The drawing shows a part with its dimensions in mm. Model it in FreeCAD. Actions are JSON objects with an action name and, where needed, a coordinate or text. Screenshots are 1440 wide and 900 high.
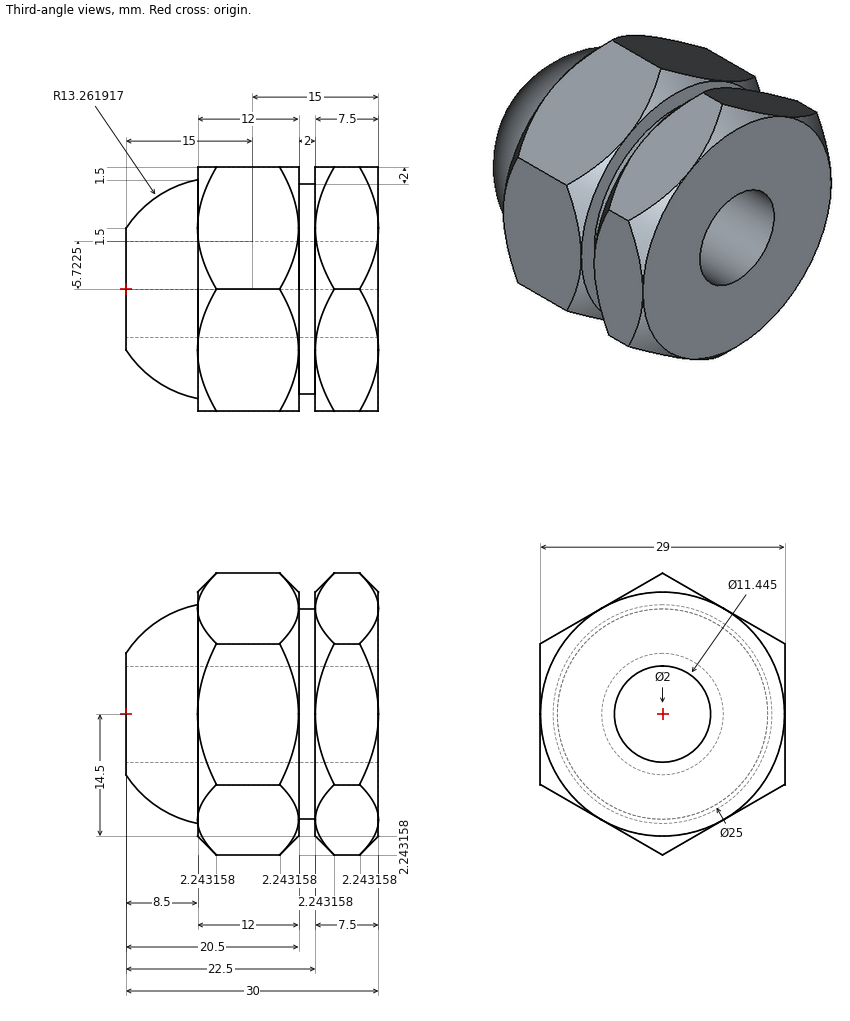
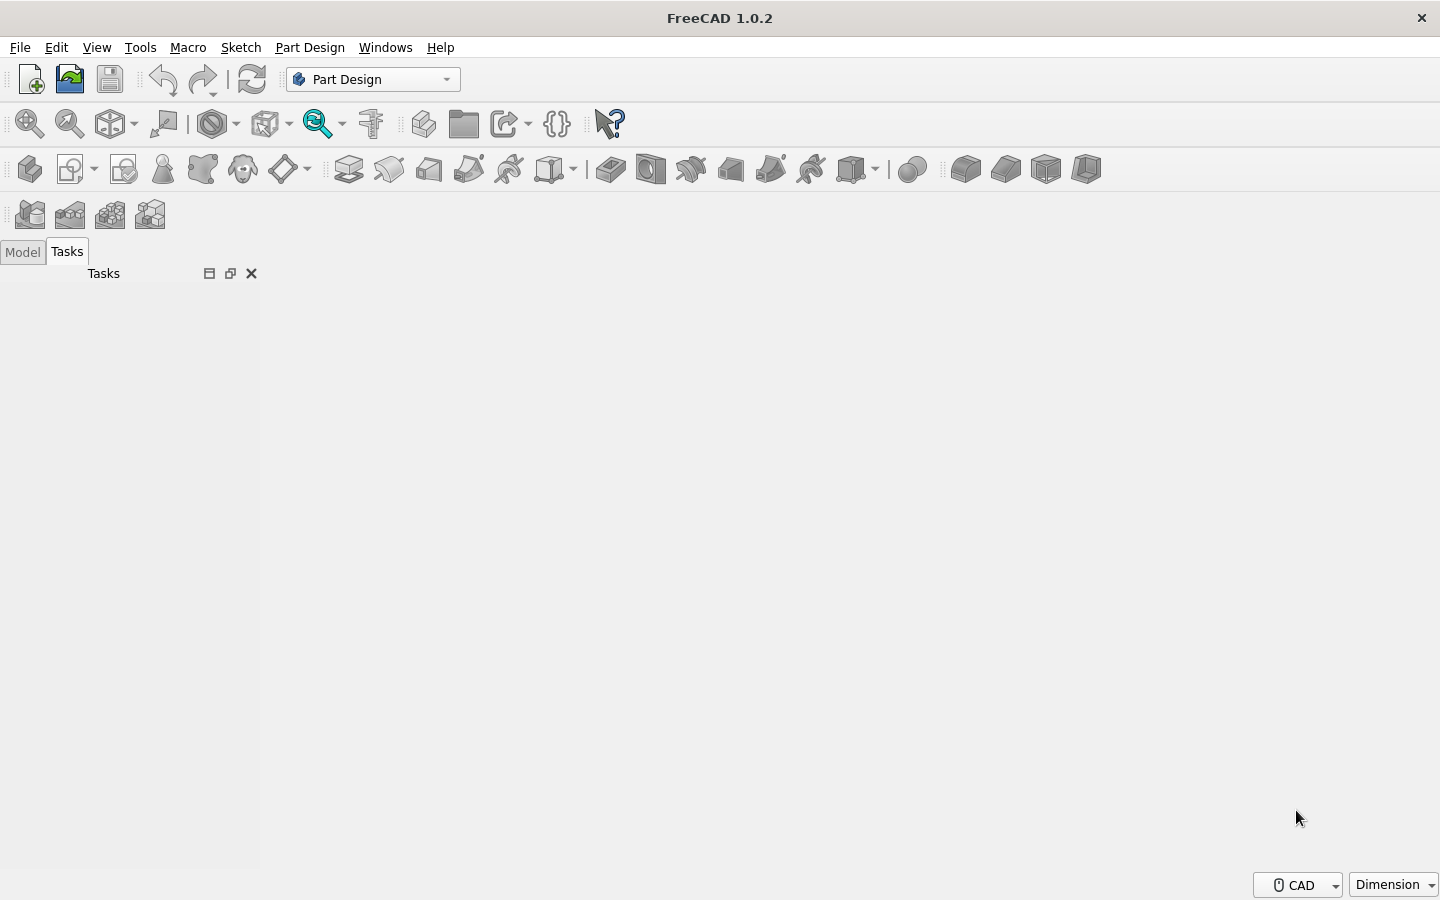
{"action": "left_click", "coordinate": [30, 80]}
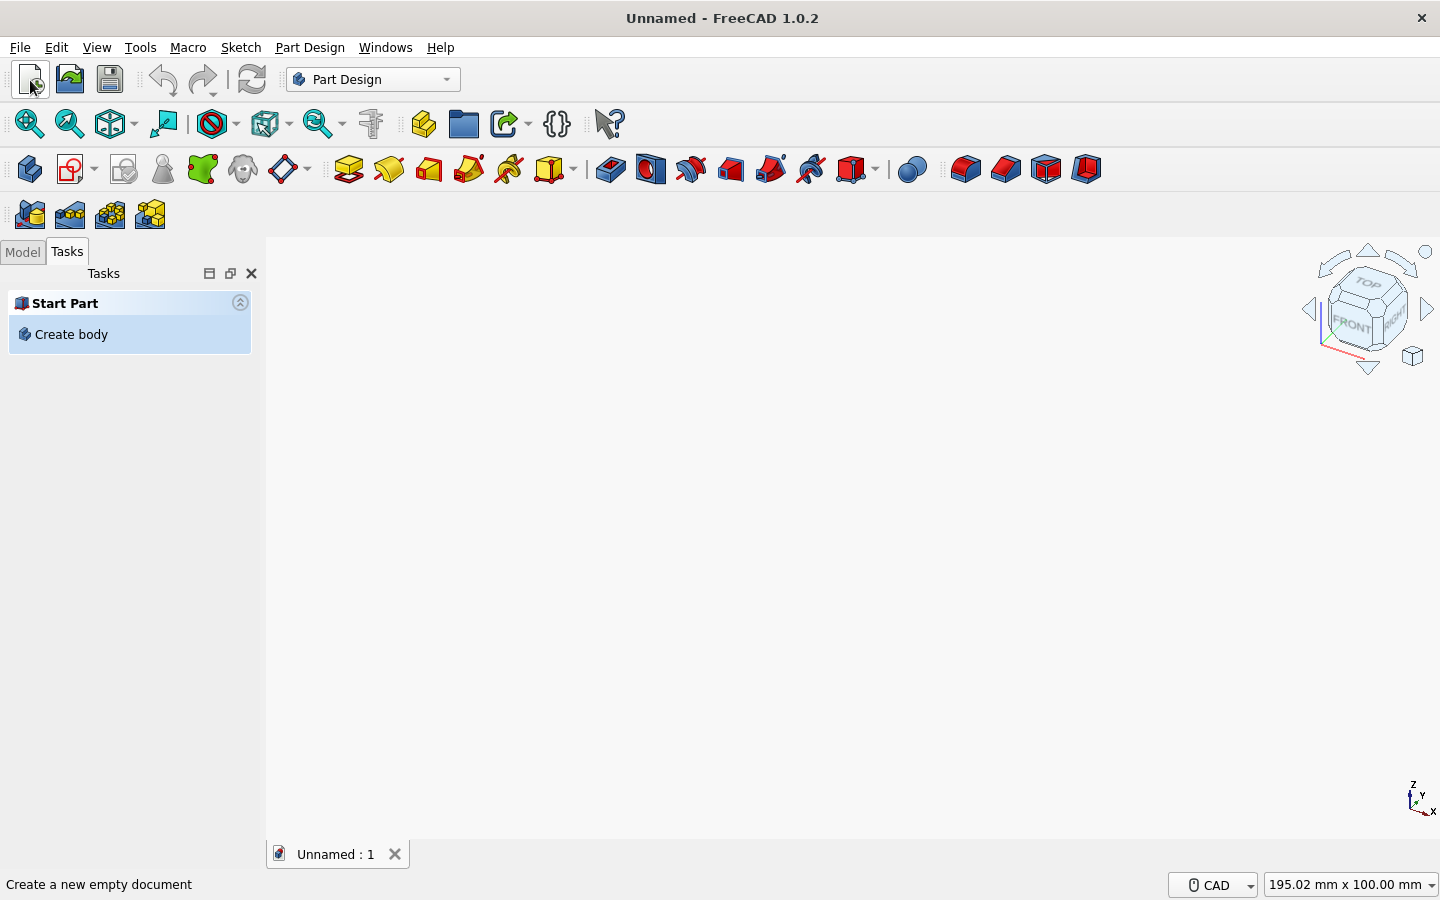
{"action": "left_click", "coordinate": [70, 170]}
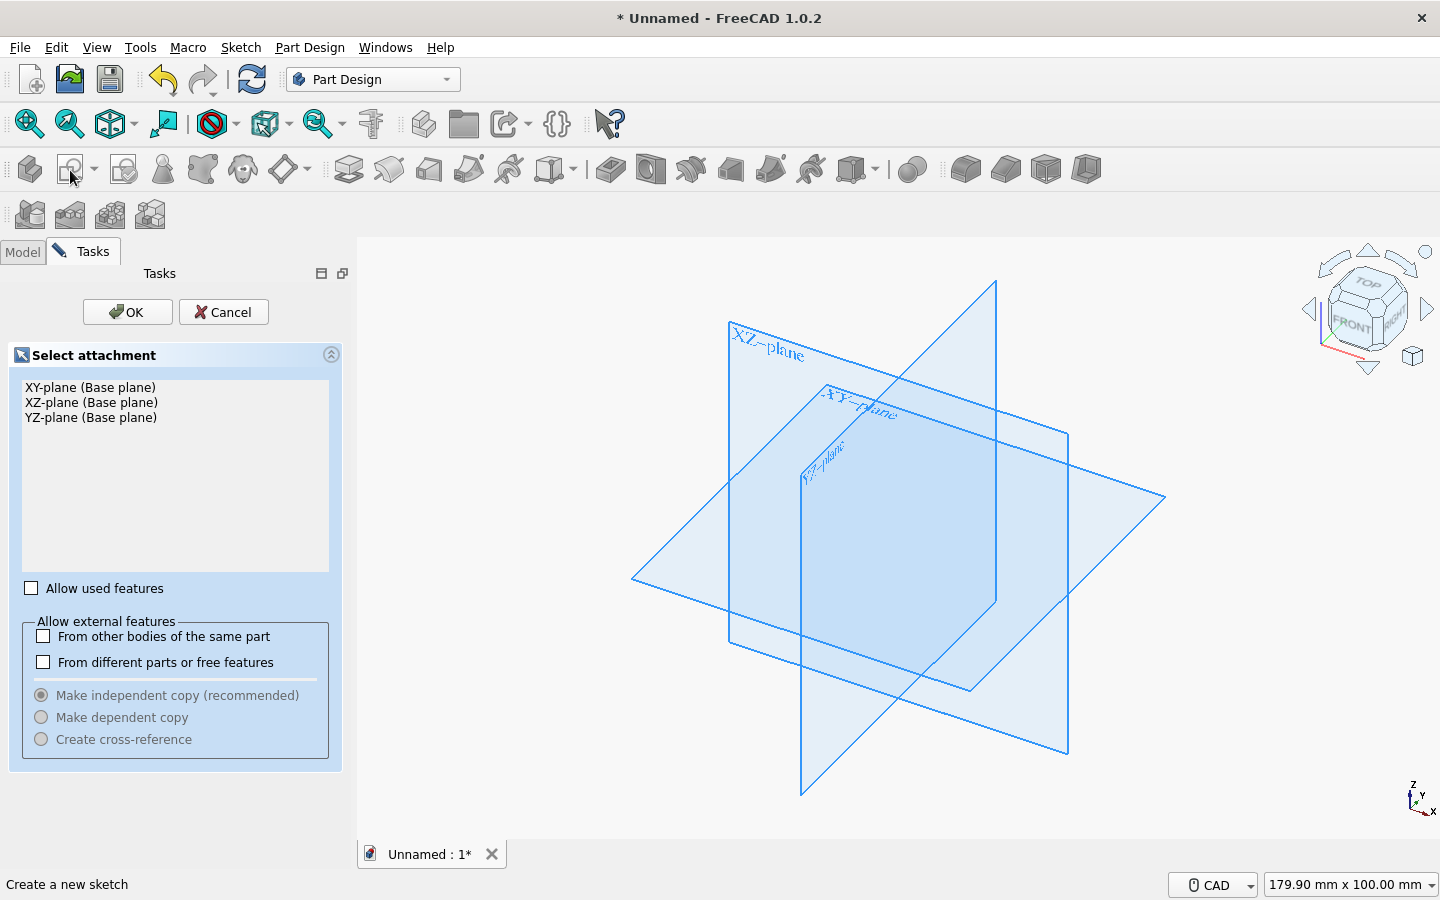
{"action": "left_click", "coordinate": [82, 388]}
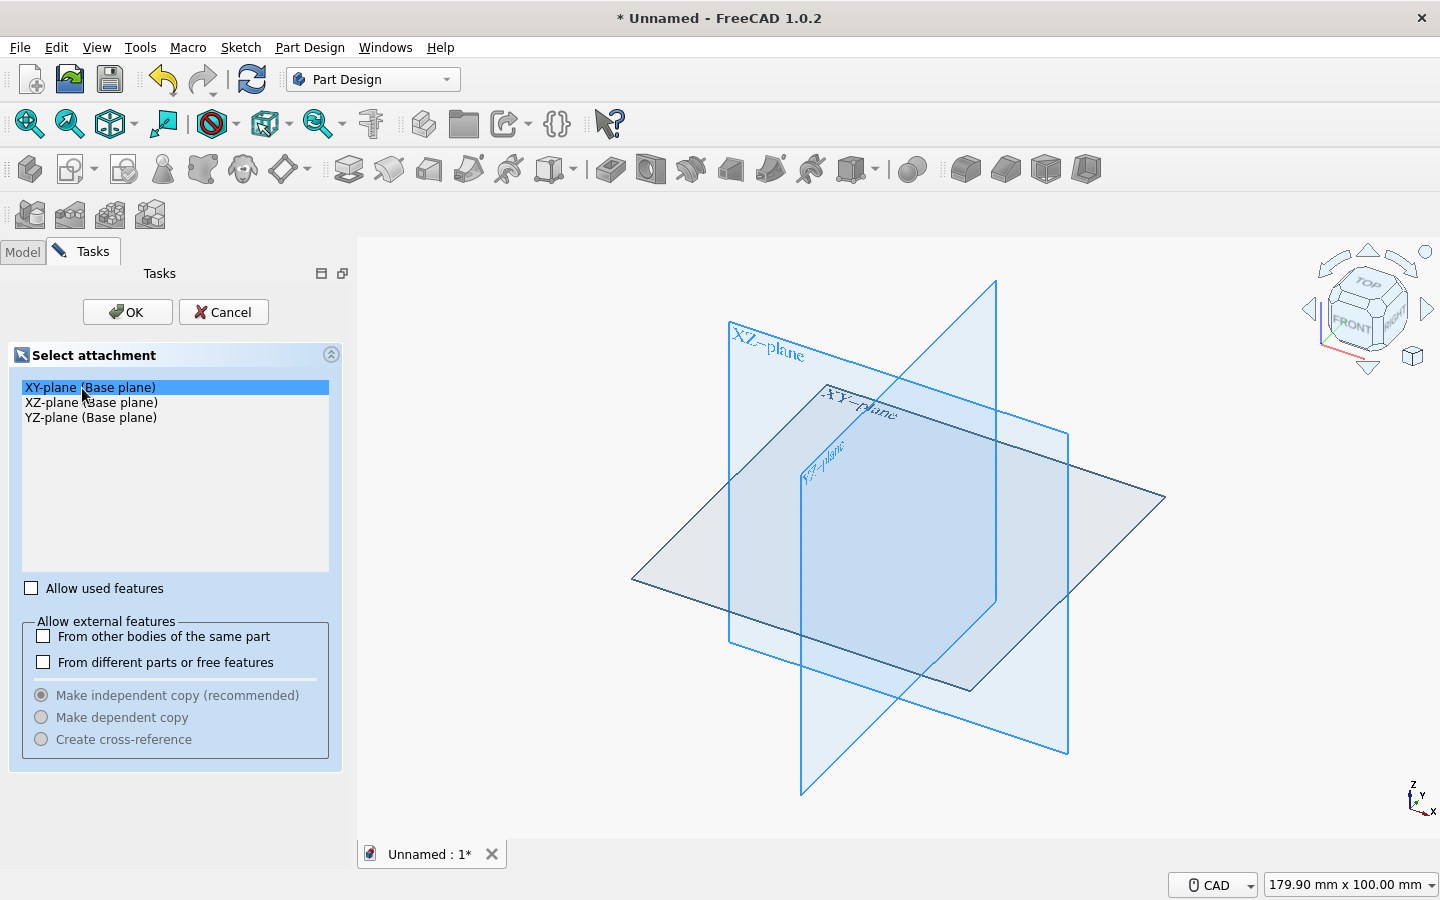
{"action": "left_click", "coordinate": [128, 312]}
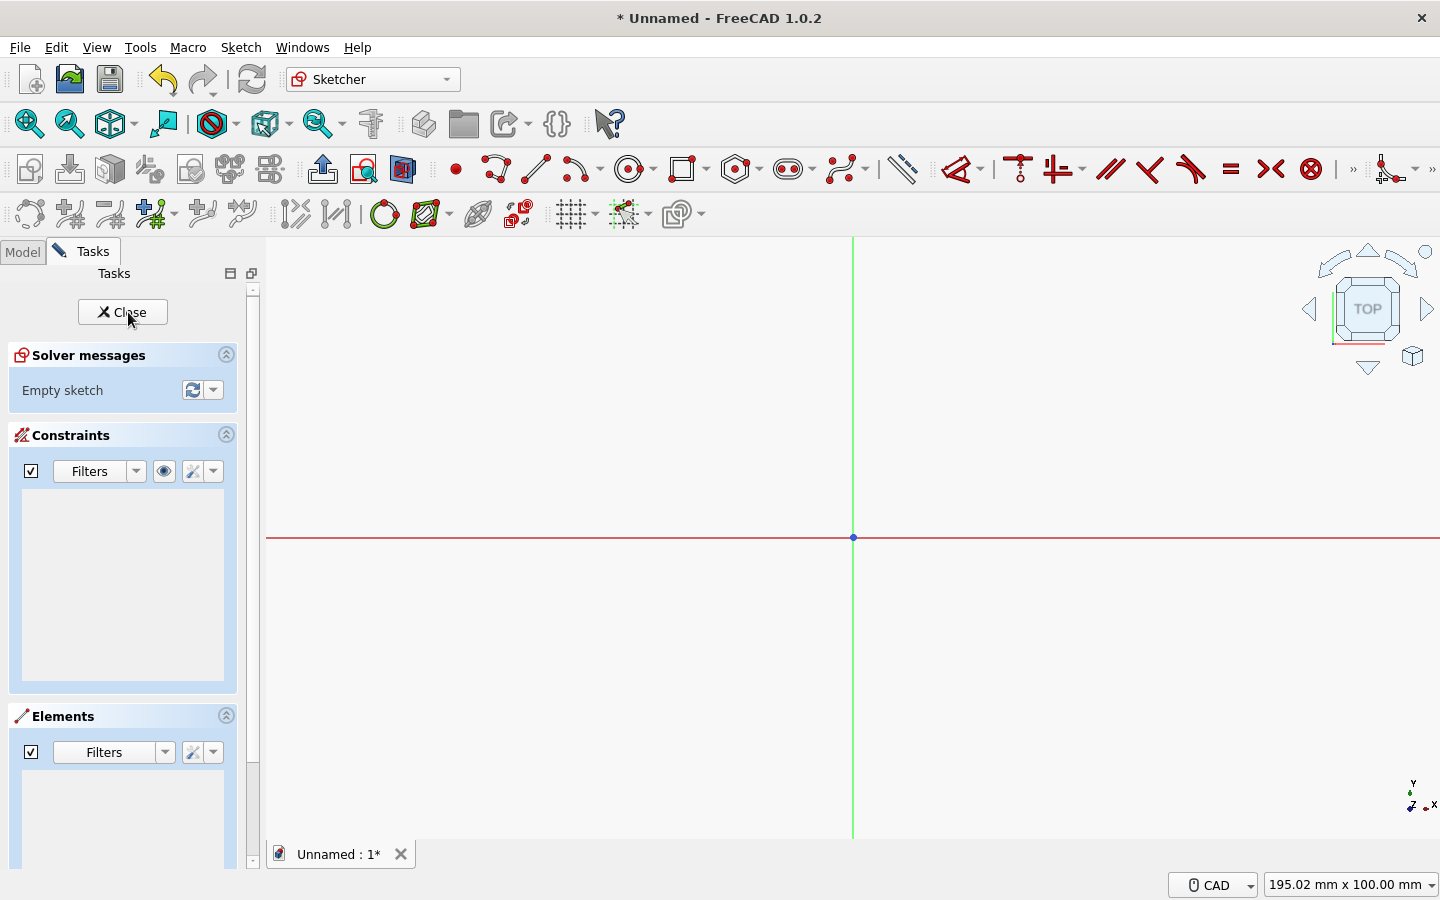
{"action": "scroll", "coordinate": [995, 480], "scroll_direction": "up", "scroll_amount": 7}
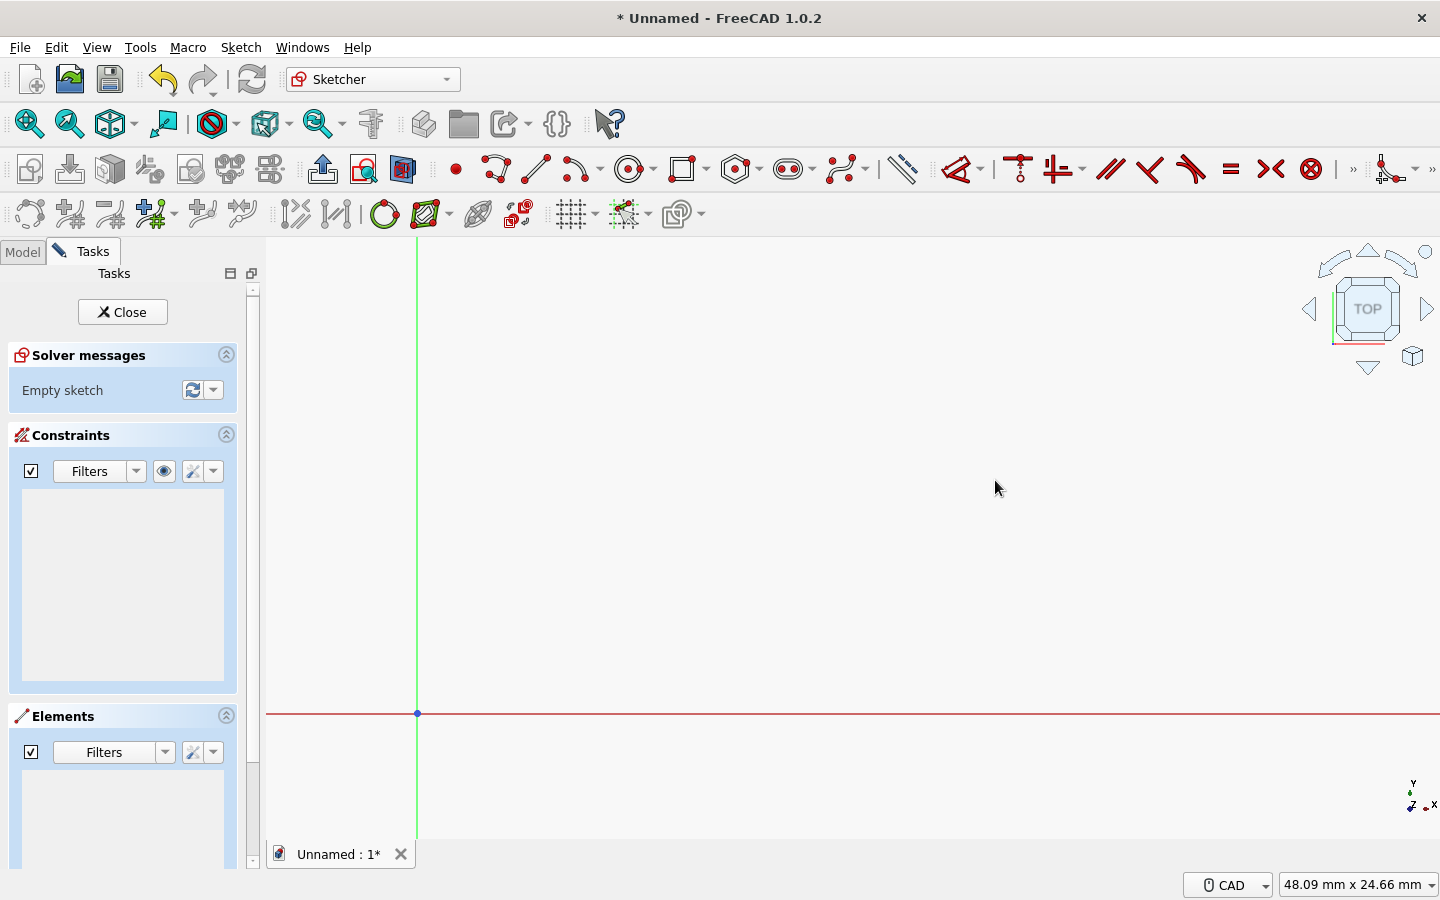
{"action": "left_click", "coordinate": [496, 170]}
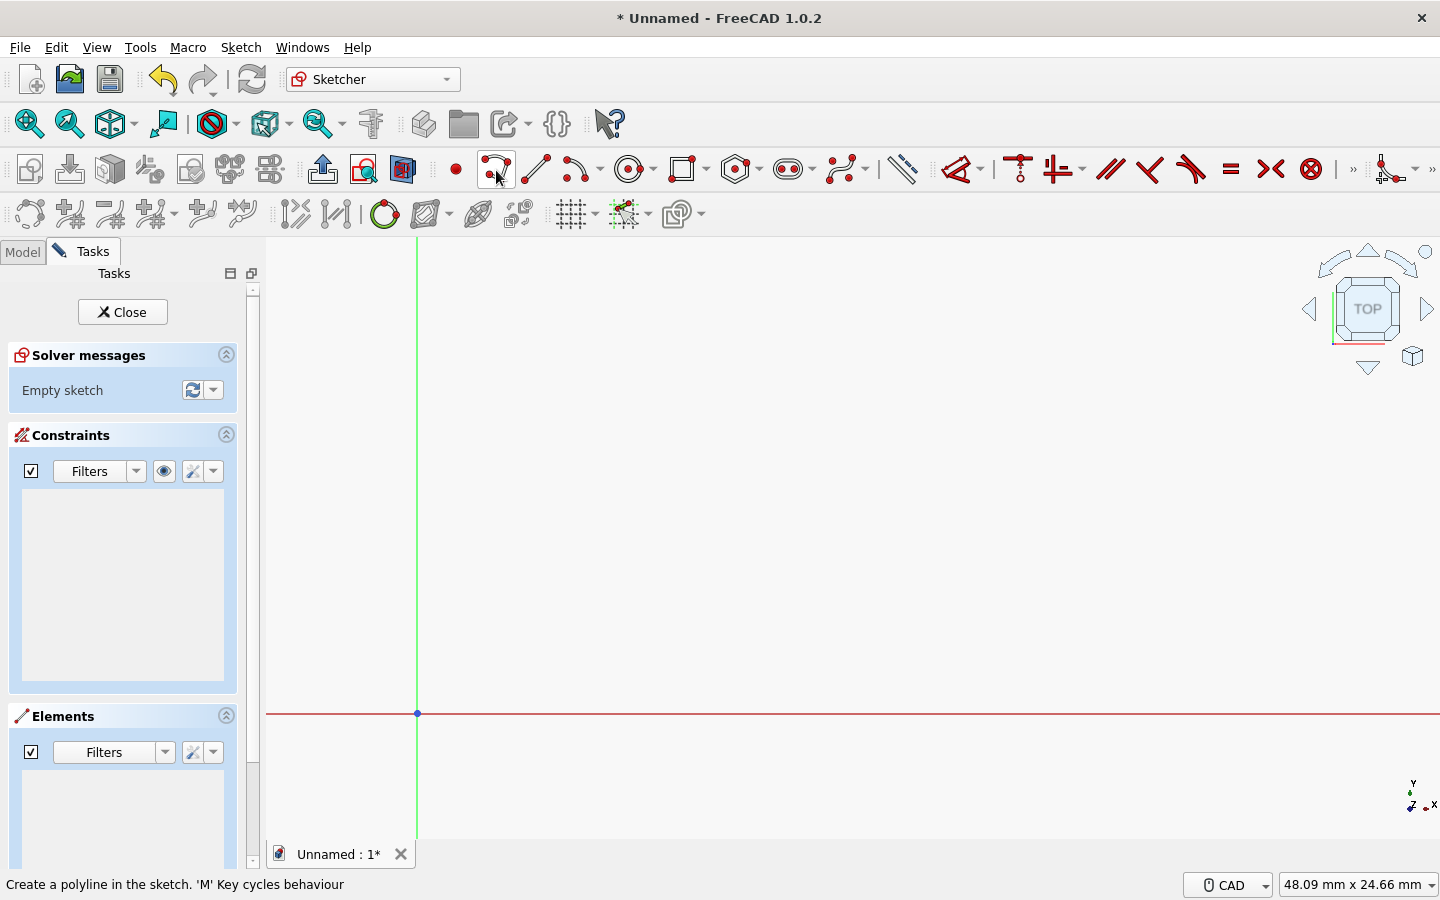
{"action": "left_click", "coordinate": [417, 538]}
{"action": "left_click", "coordinate": [426, 574]}
{"action": "left_click", "coordinate": [783, 574]}
{"action": "left_click", "coordinate": [783, 714]}
{"action": "left_click", "coordinate": [1150, 705]}
{"action": "left_click", "coordinate": [1150, 360]}
{"action": "left_click", "coordinate": [967, 360]}
{"action": "left_click", "coordinate": [967, 409]}
{"action": "left_click", "coordinate": [918, 409]}
{"action": "left_click", "coordinate": [918, 360]}
{"action": "left_click", "coordinate": [625, 360]}
{"action": "left_click", "coordinate": [625, 397]}
{"action": "right_click", "coordinate": [625, 397]}